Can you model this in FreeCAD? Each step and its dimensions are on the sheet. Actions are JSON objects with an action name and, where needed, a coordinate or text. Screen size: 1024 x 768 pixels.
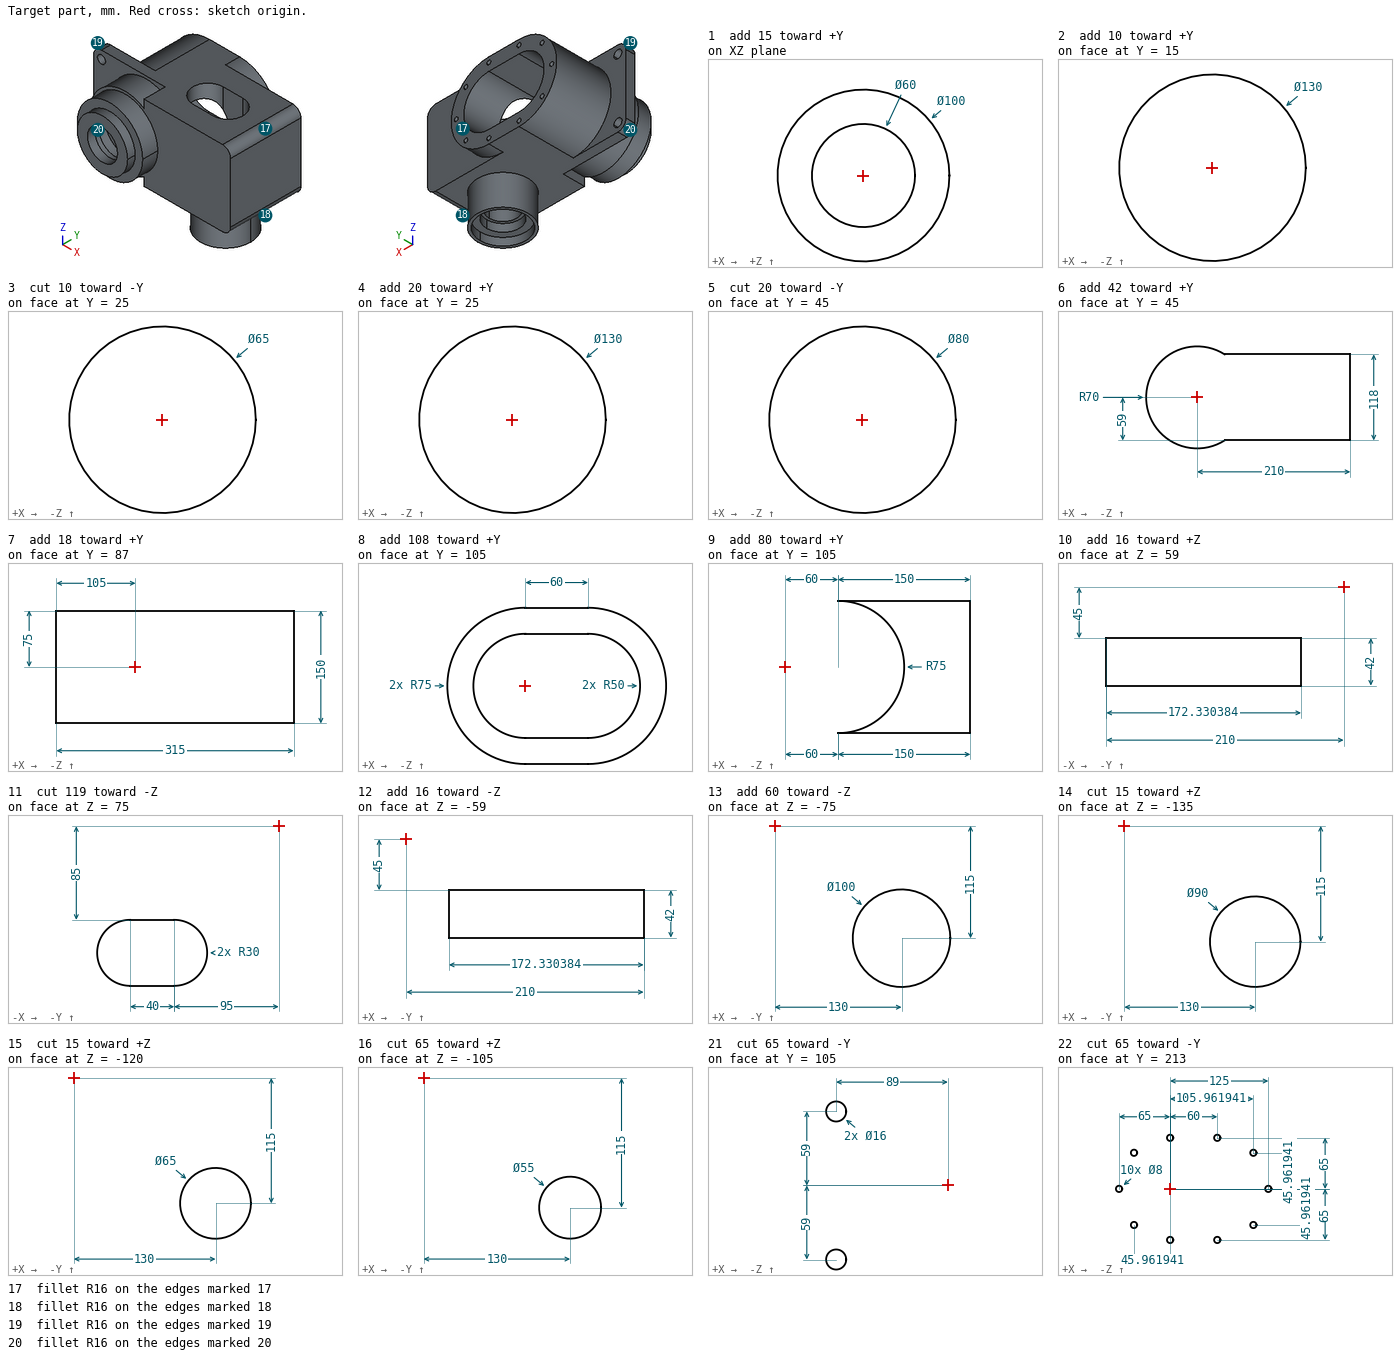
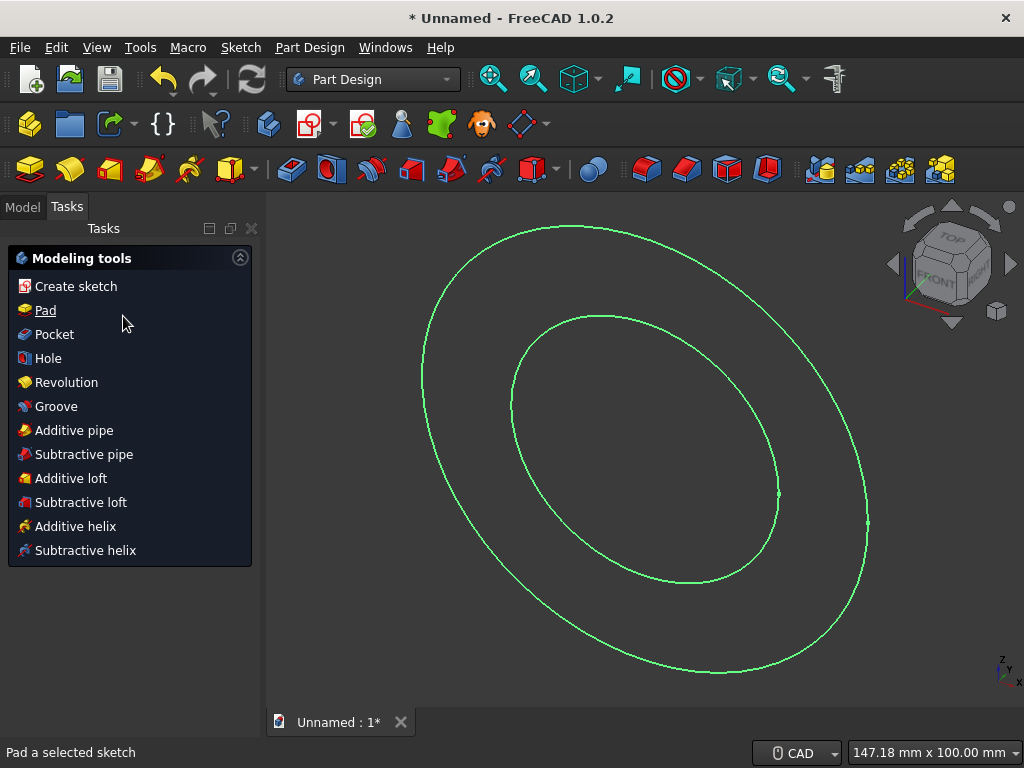
{"action": "left_click", "coordinate": [30, 170]}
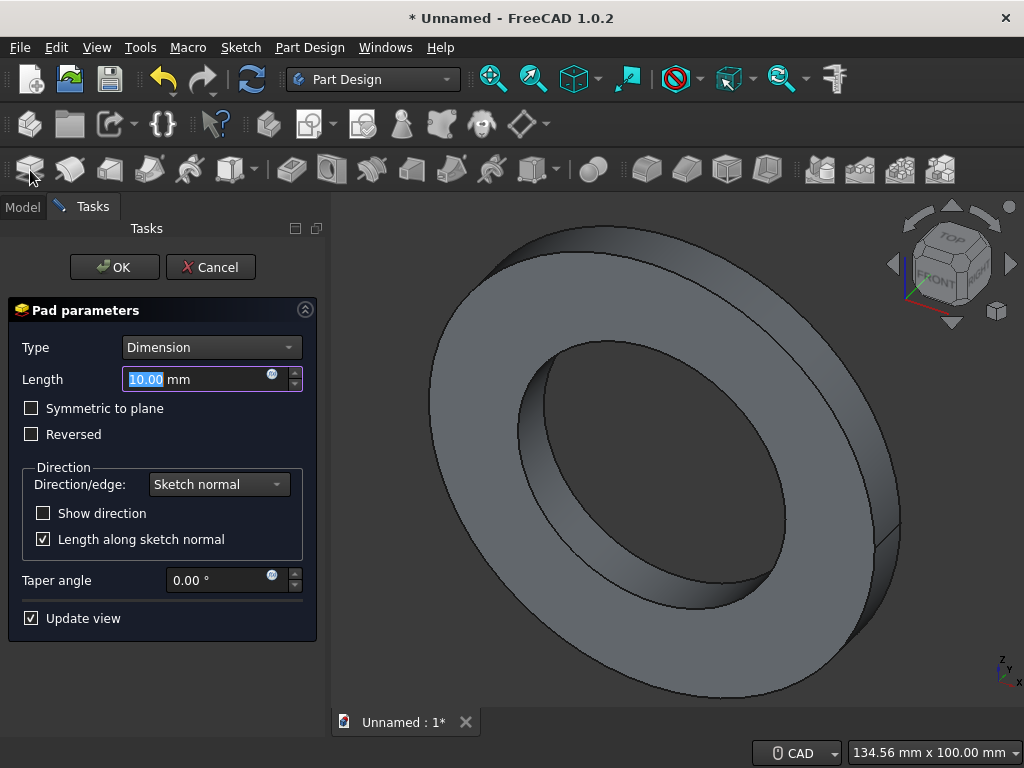
{"action": "type", "text": "15"}
{"action": "key", "text": "Tab"}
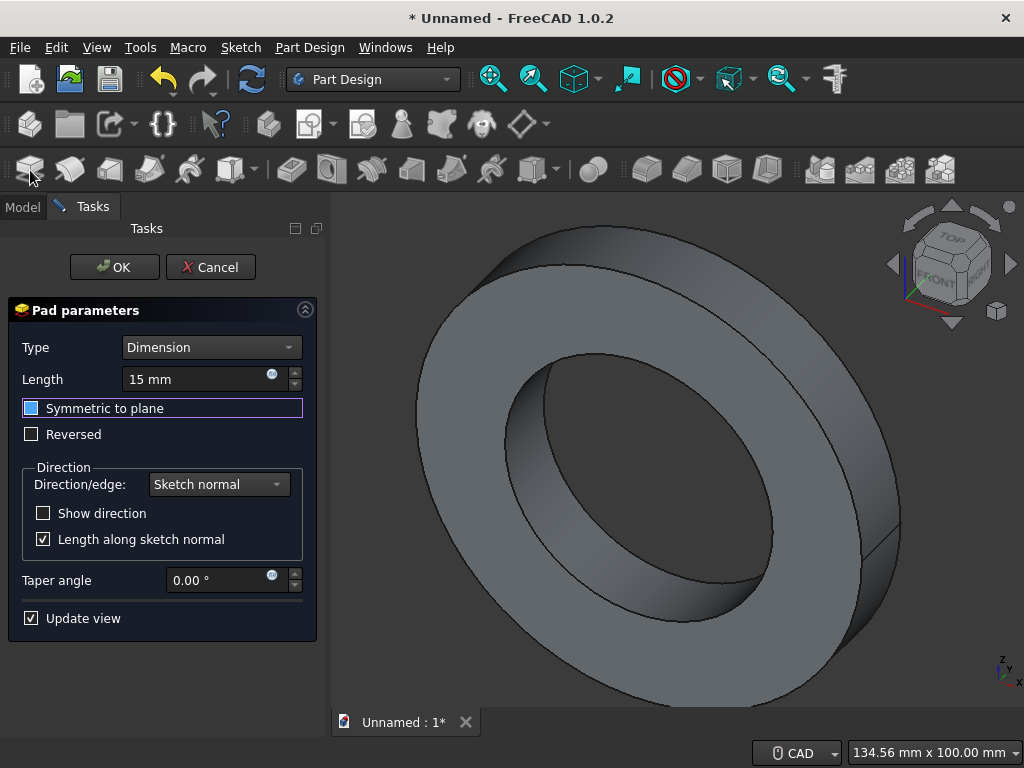
{"action": "left_click", "coordinate": [30, 434]}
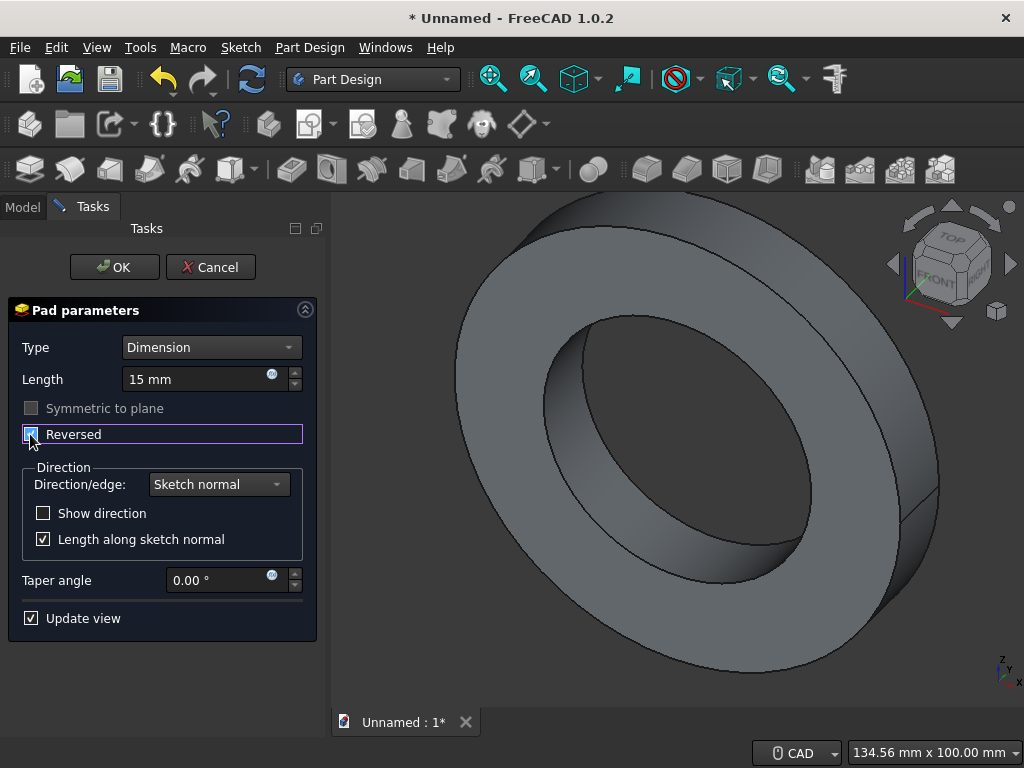
{"action": "left_click", "coordinate": [115, 267]}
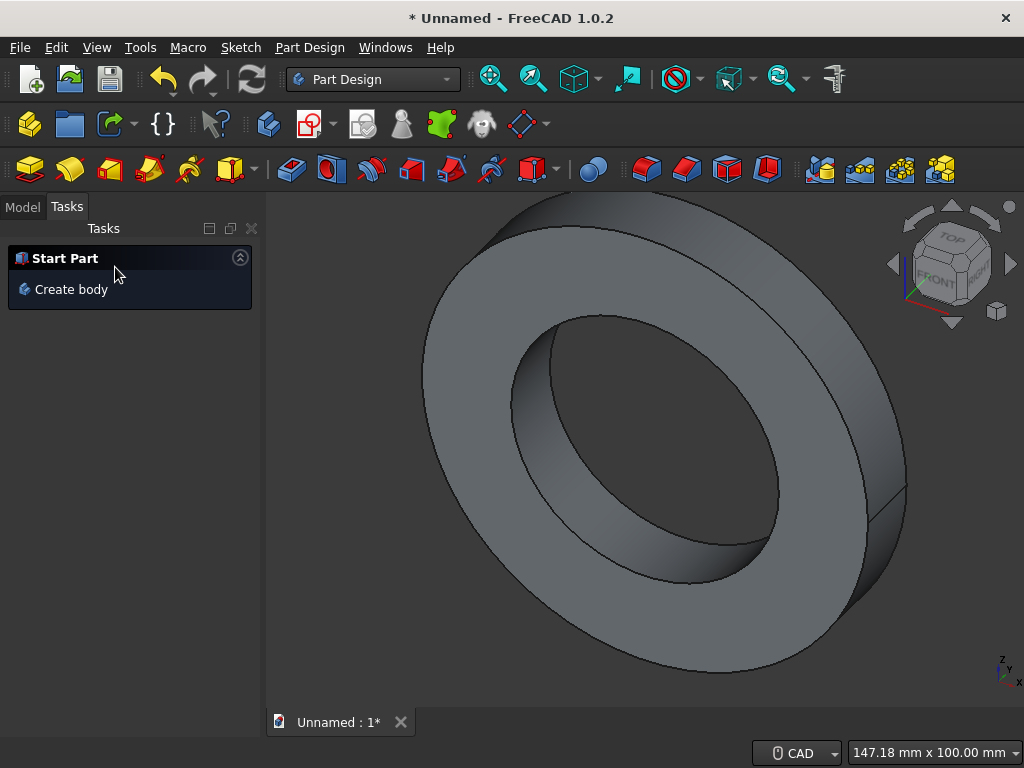
{"action": "left_click", "coordinate": [494, 80]}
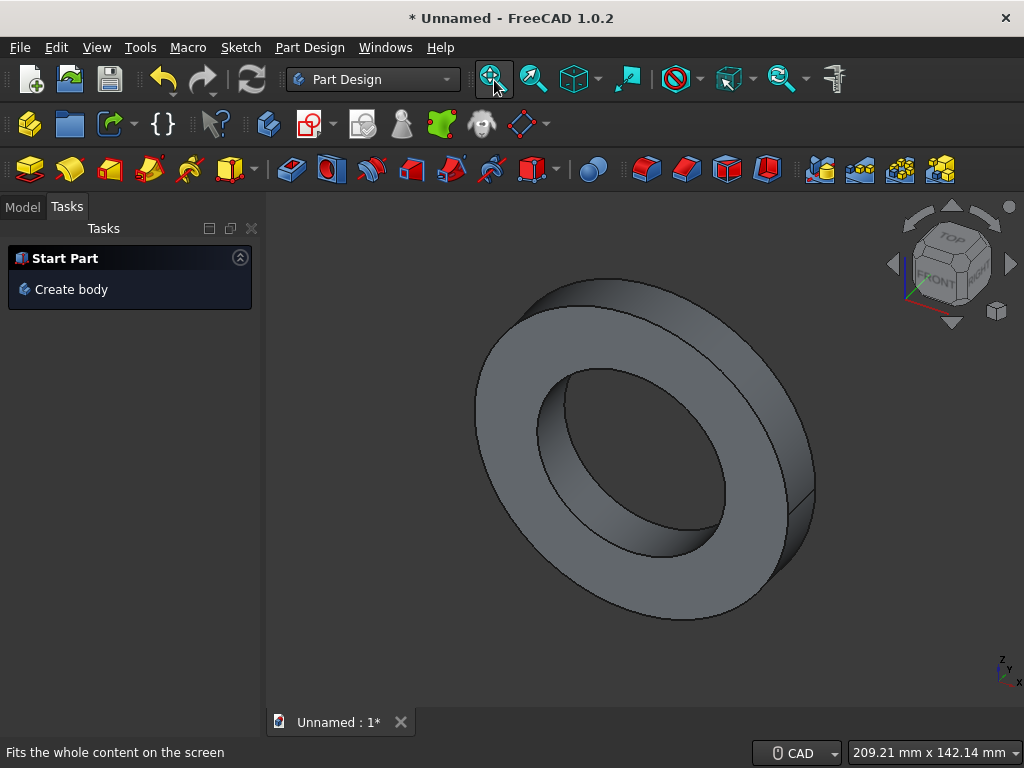
{"action": "key", "text": "4"}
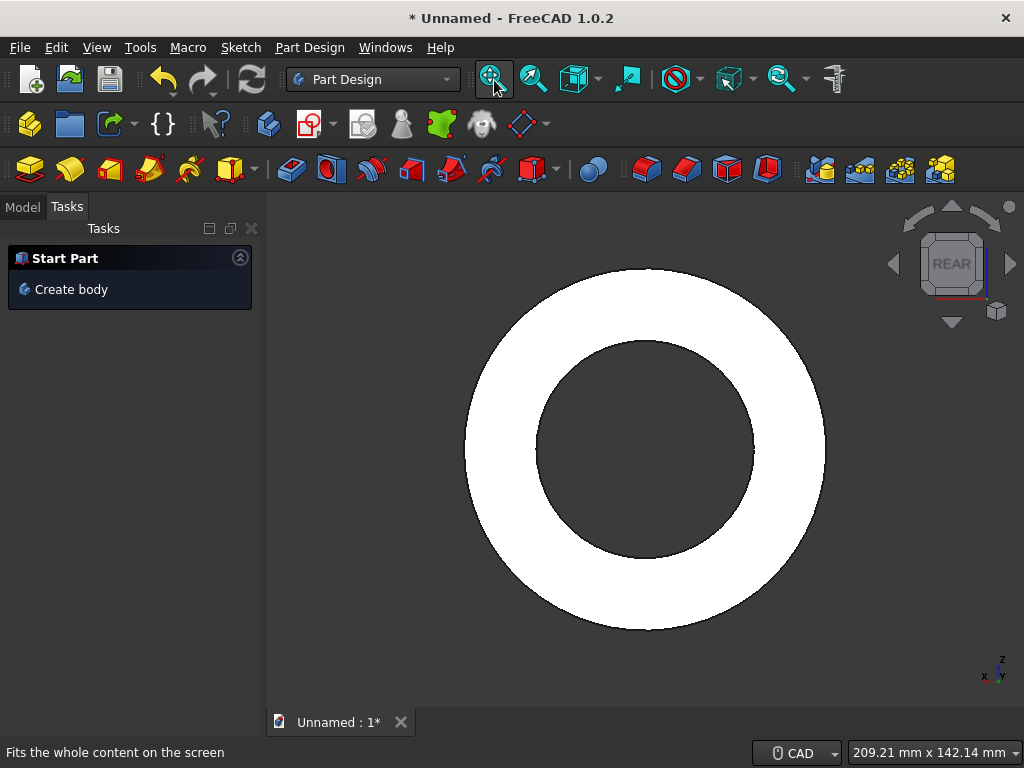
{"action": "left_click", "coordinate": [542, 345]}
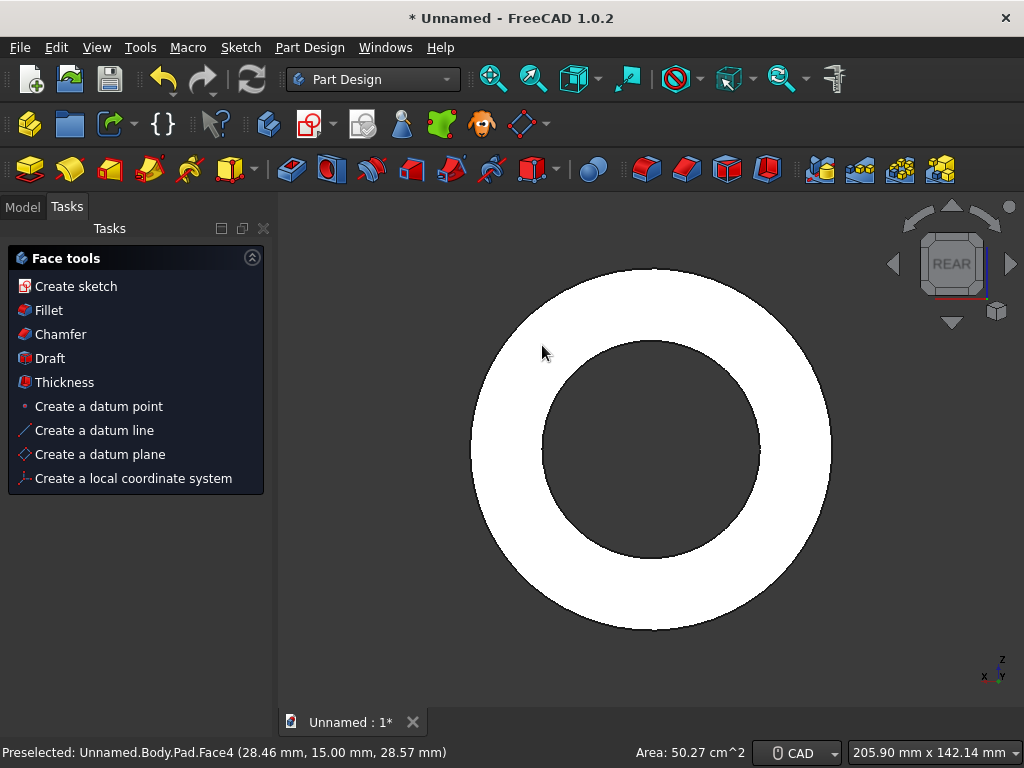
{"action": "left_click", "coordinate": [310, 124]}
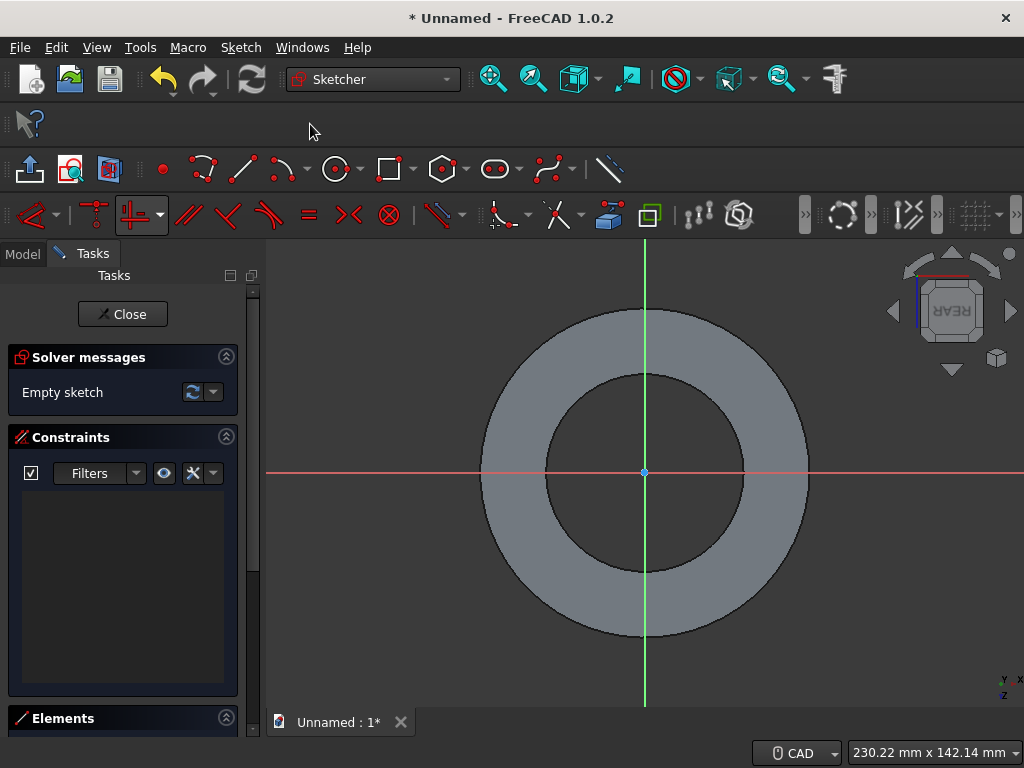
{"action": "scroll", "coordinate": [437, 473], "scroll_direction": "down", "scroll_amount": 2}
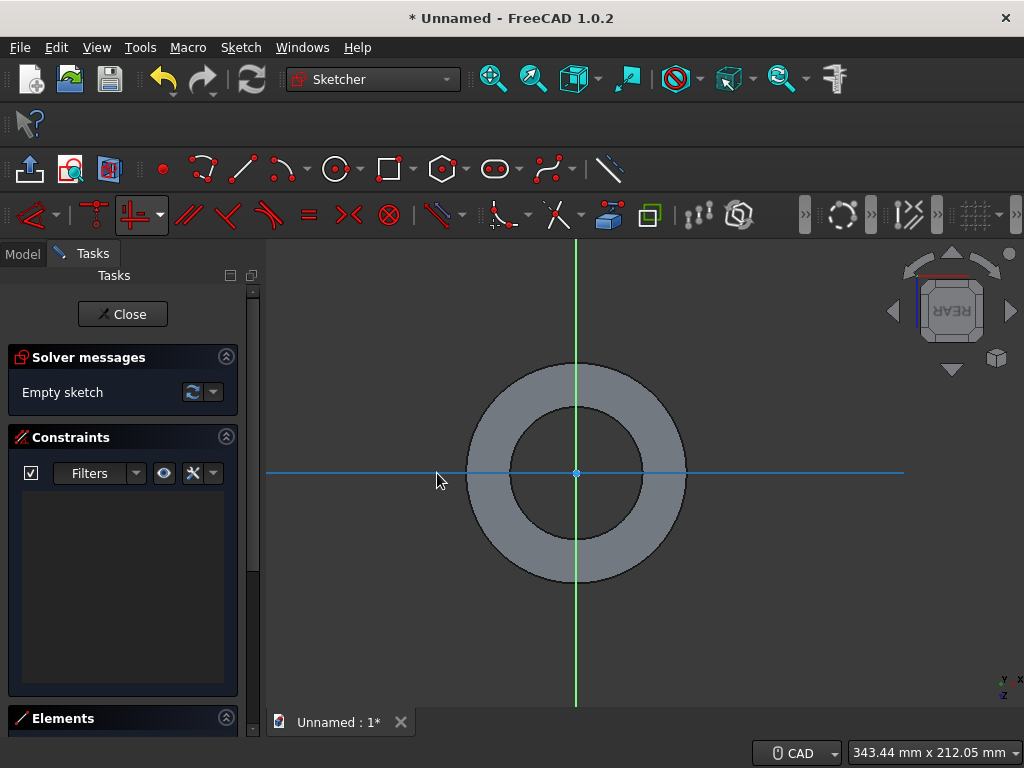
{"action": "left_click", "coordinate": [336, 170]}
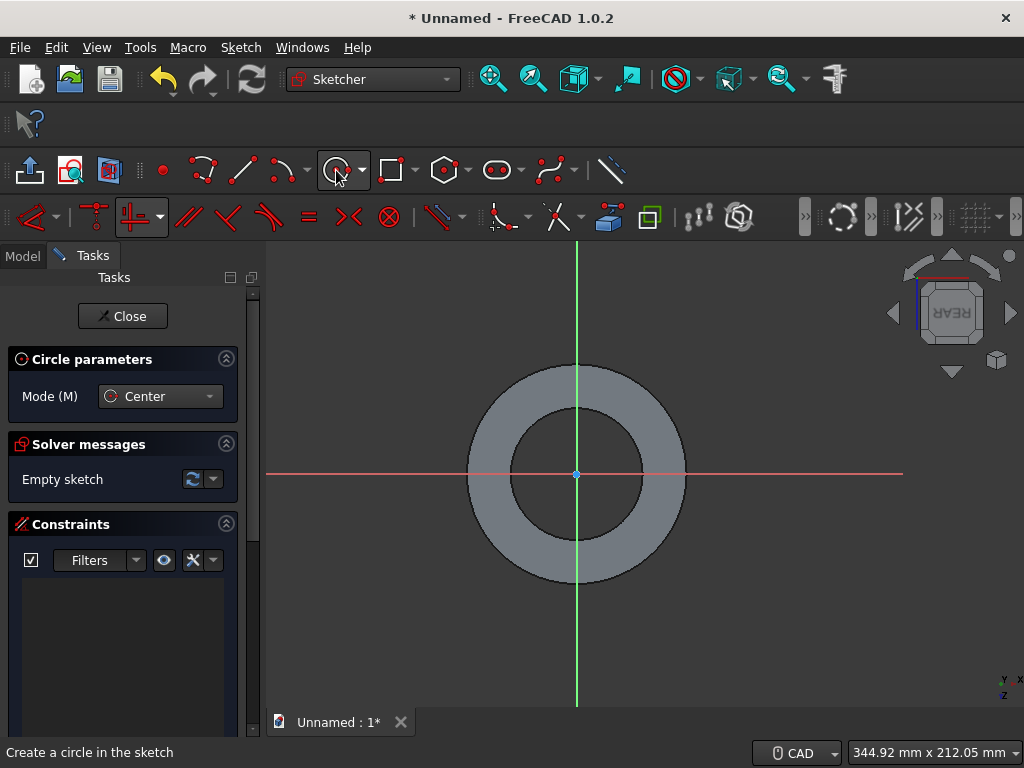
{"action": "left_click", "coordinate": [577, 474]}
{"action": "mouse_move", "coordinate": [678, 373]}